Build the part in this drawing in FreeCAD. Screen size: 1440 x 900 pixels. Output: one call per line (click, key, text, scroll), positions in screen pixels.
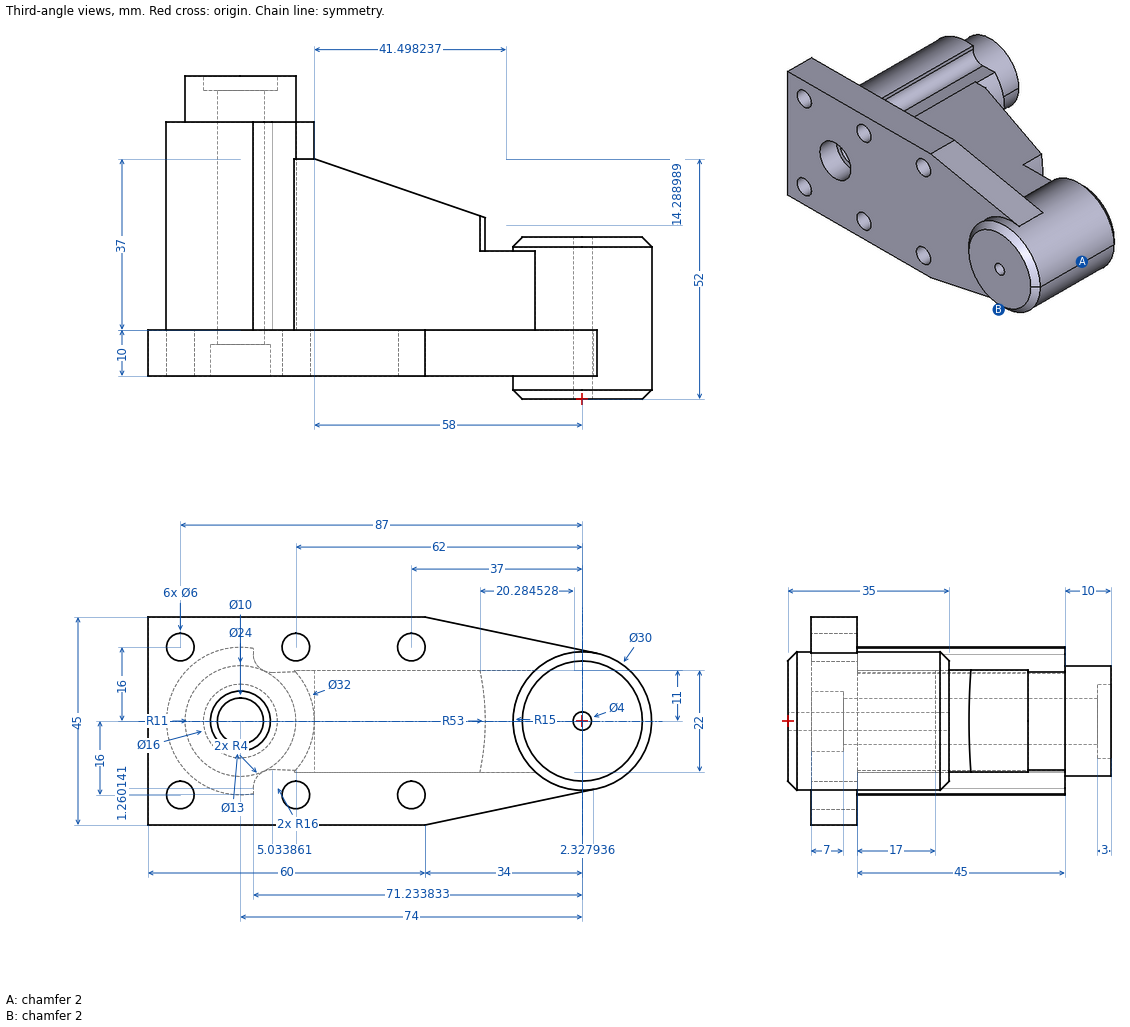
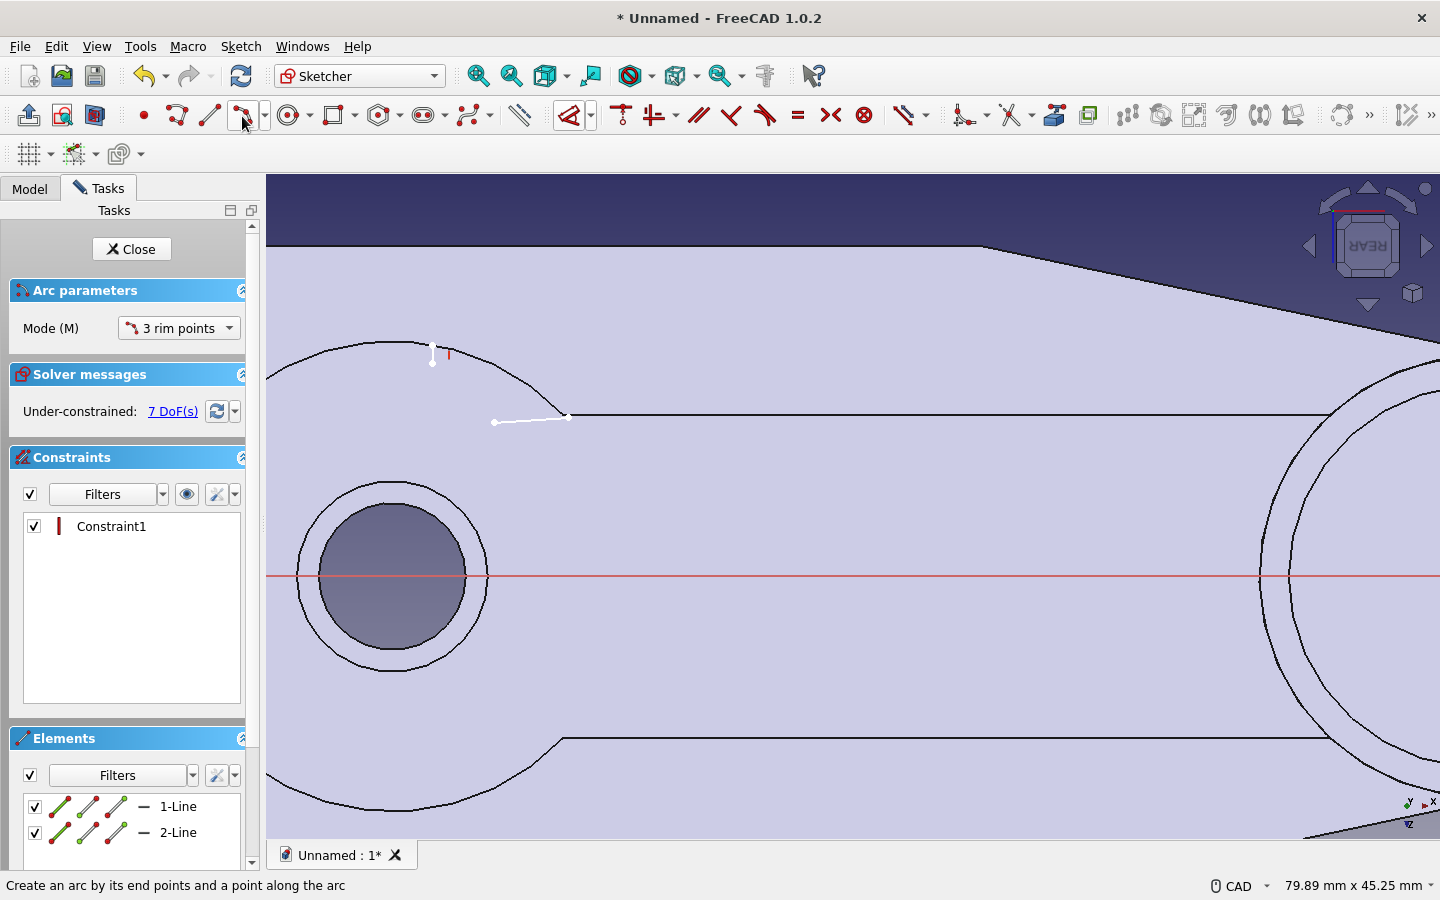
scroll(433, 363, up, 3)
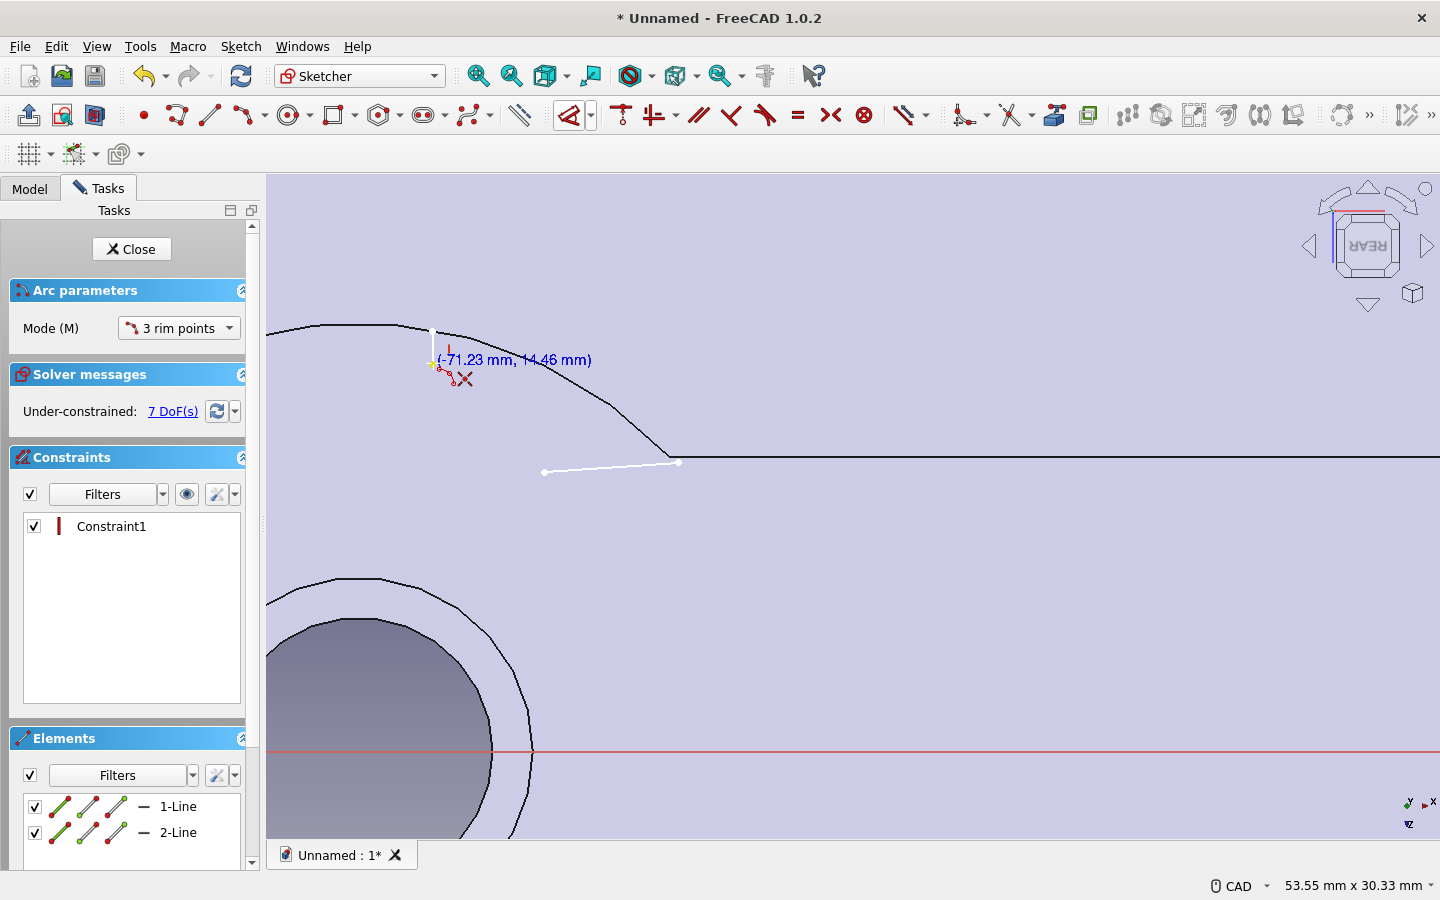
click(433, 365)
click(544, 472)
click(465, 440)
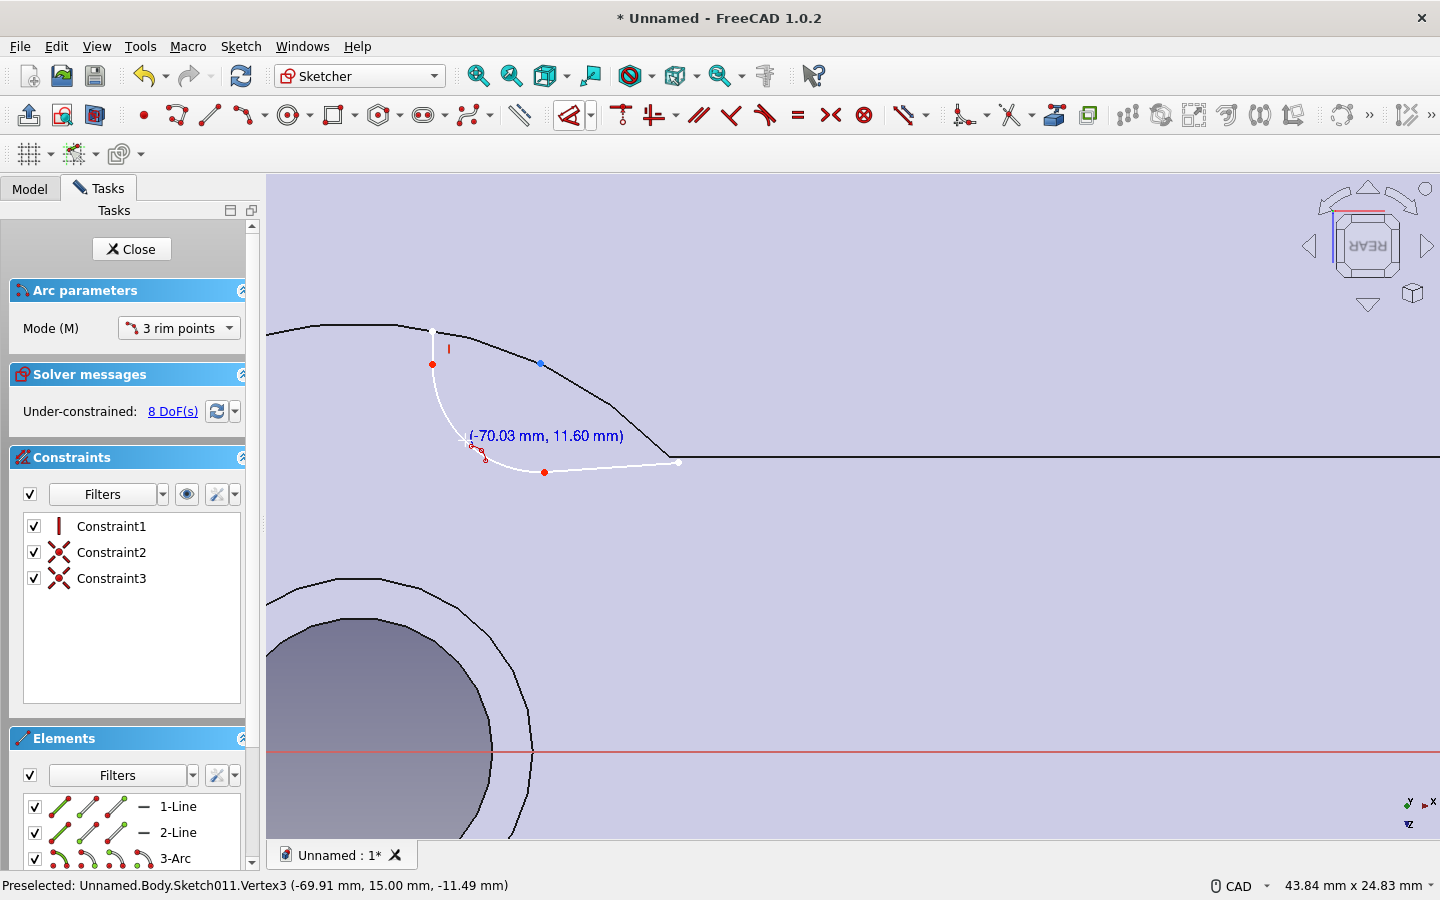
click(679, 463)
click(433, 332)
click(567, 377)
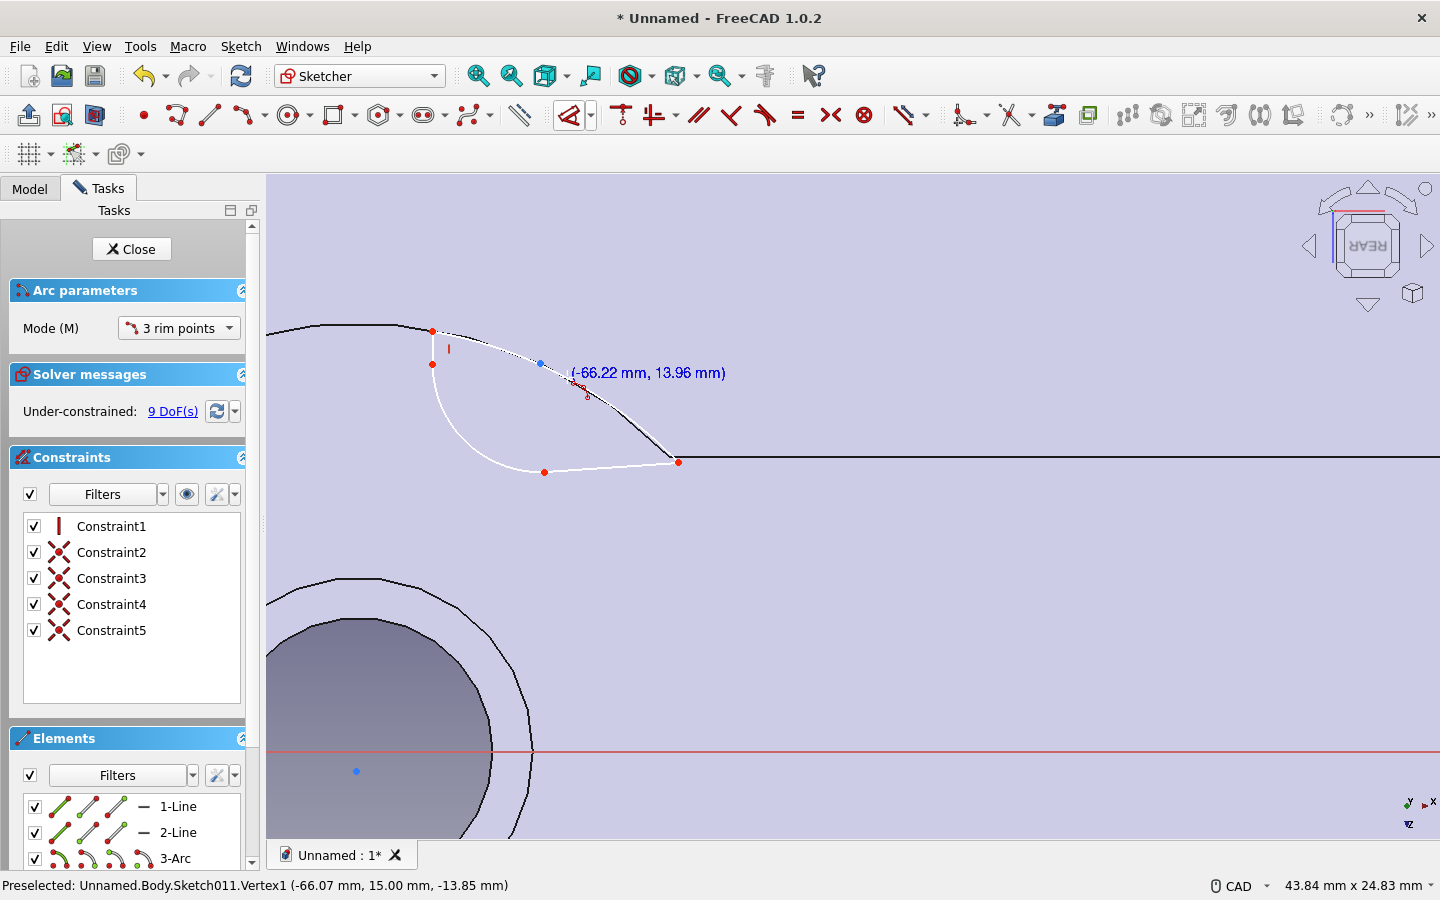
click(210, 116)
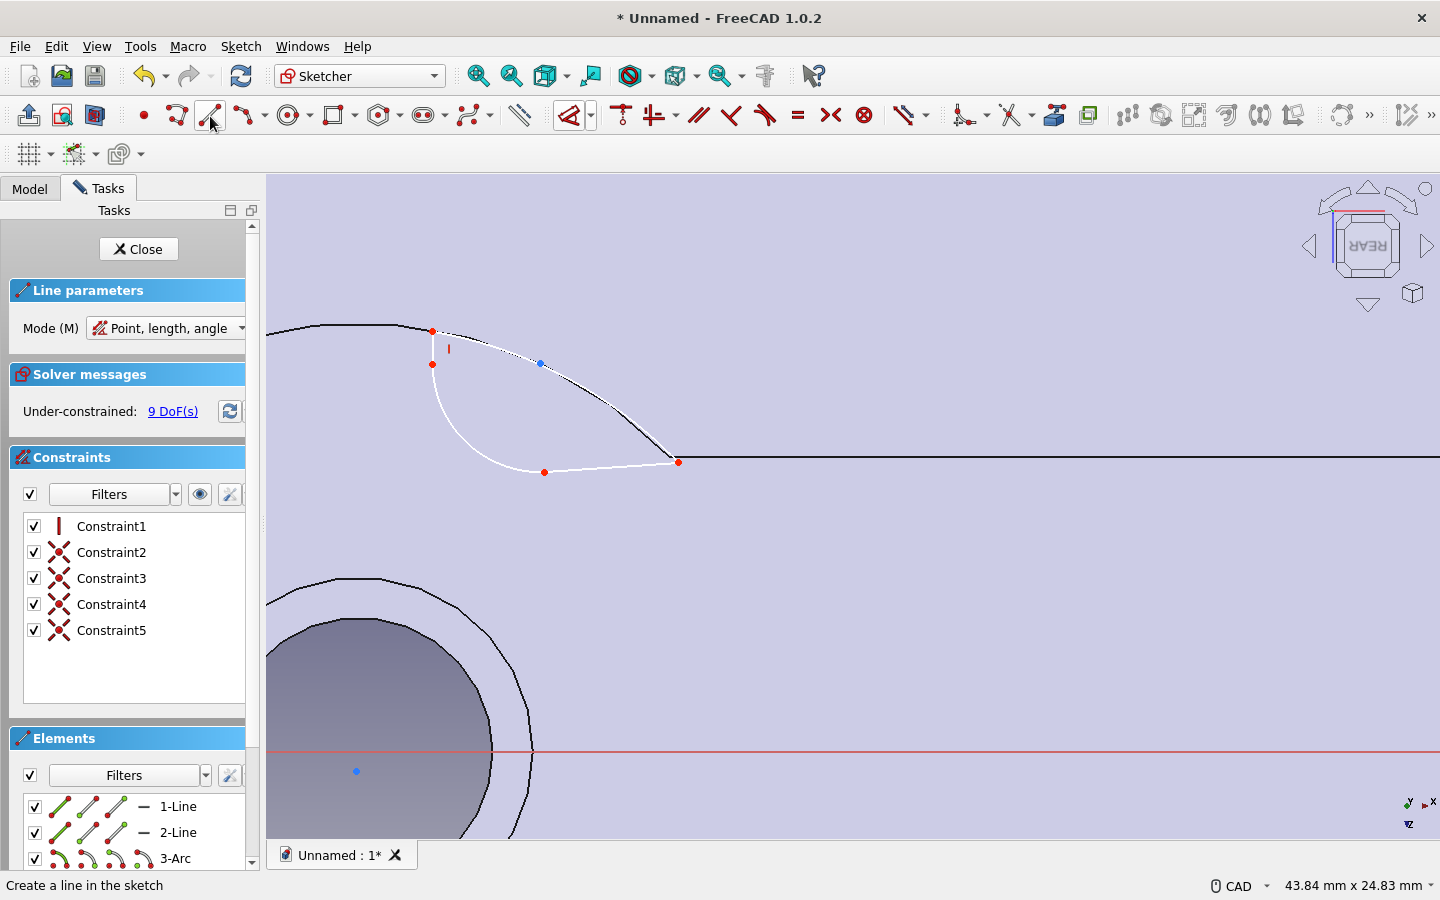
scroll(434, 364, down, 5)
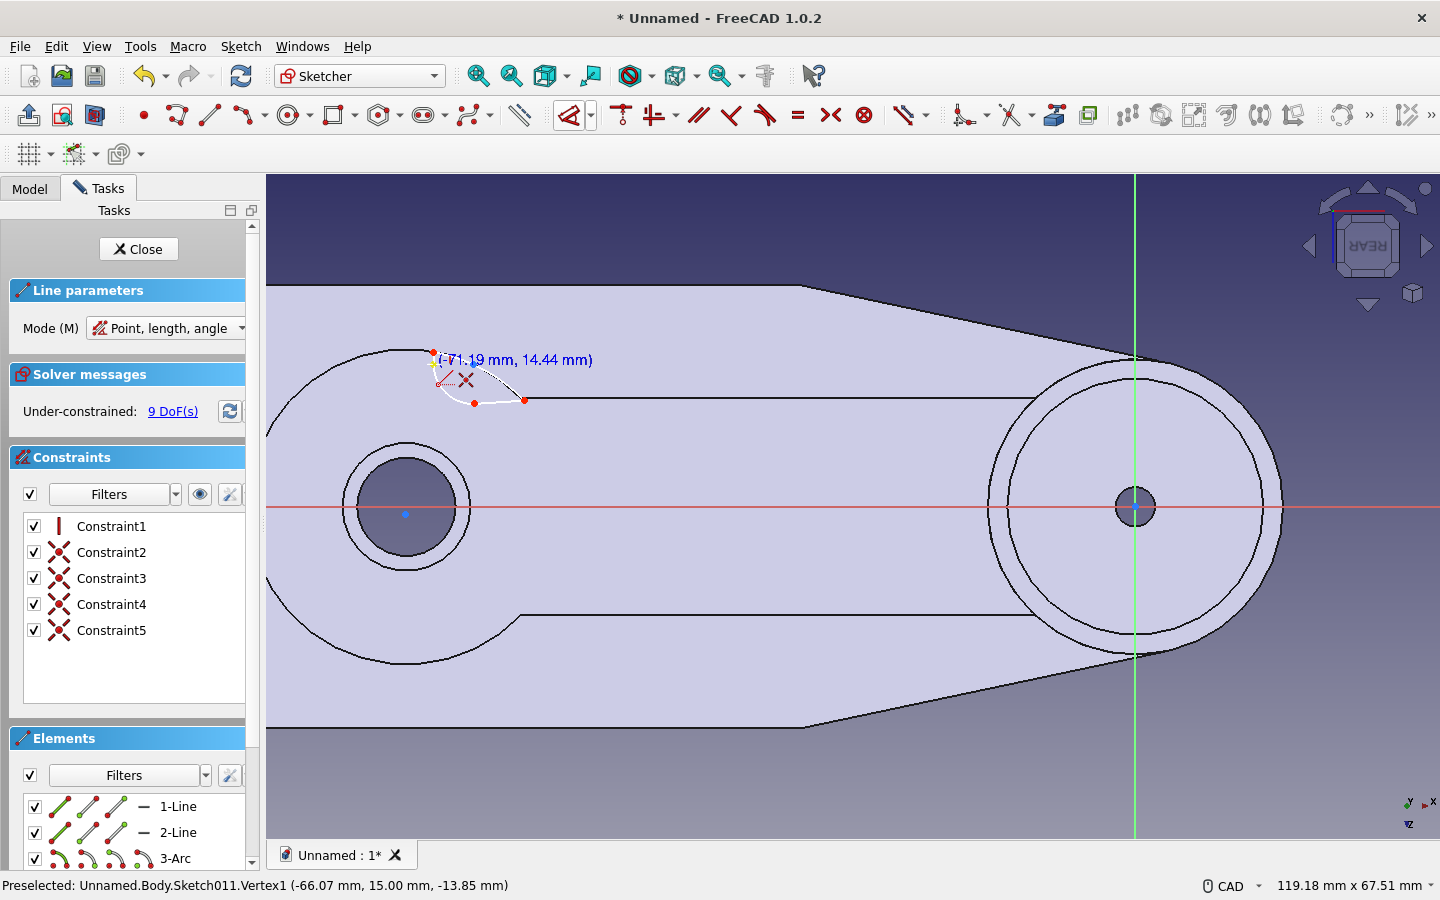
click(524, 612)
click(474, 608)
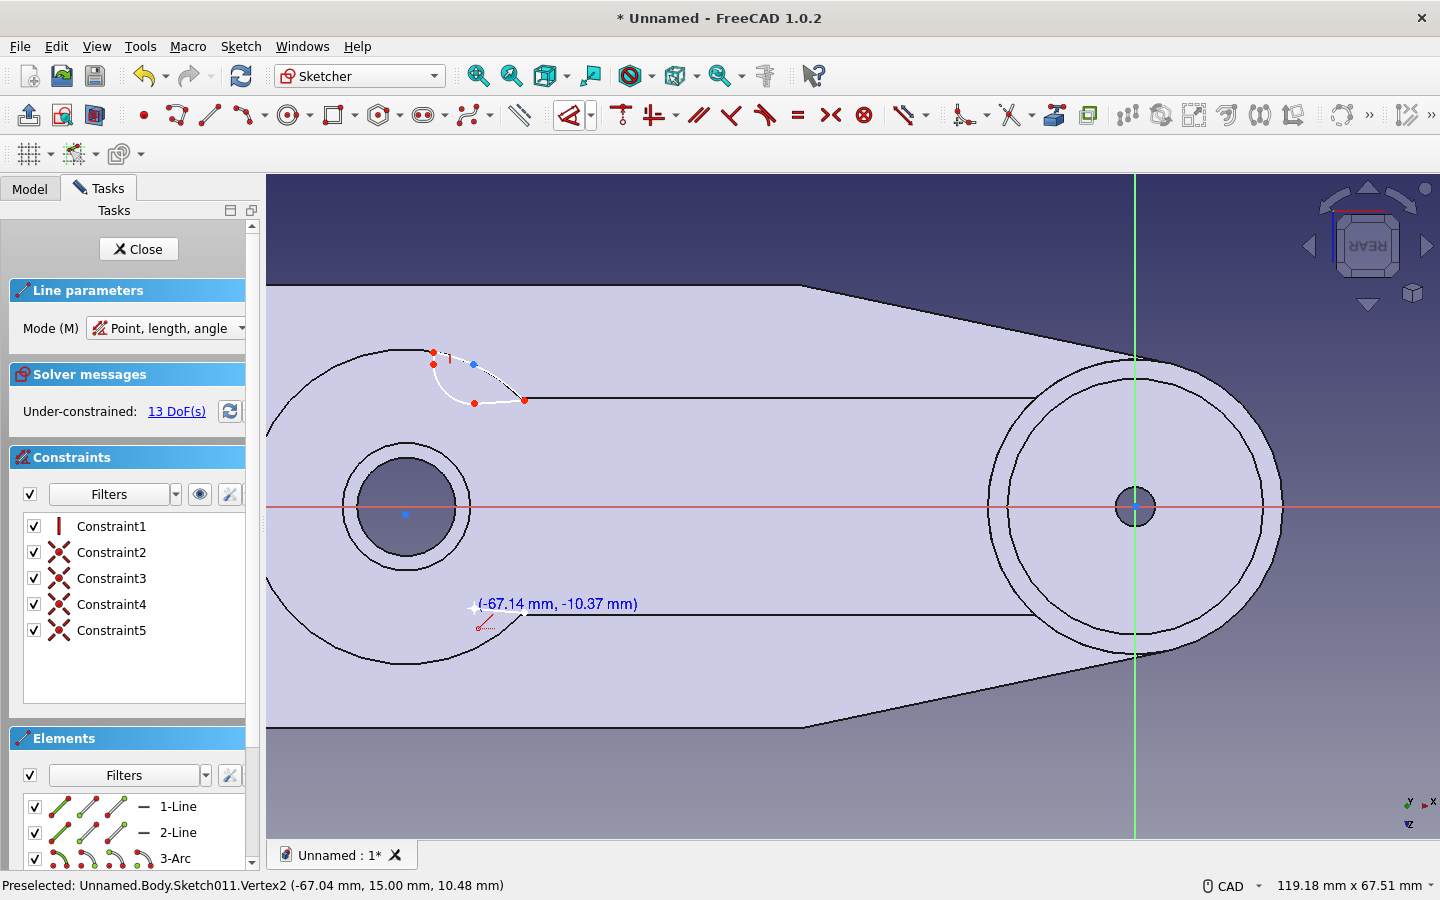
click(434, 650)